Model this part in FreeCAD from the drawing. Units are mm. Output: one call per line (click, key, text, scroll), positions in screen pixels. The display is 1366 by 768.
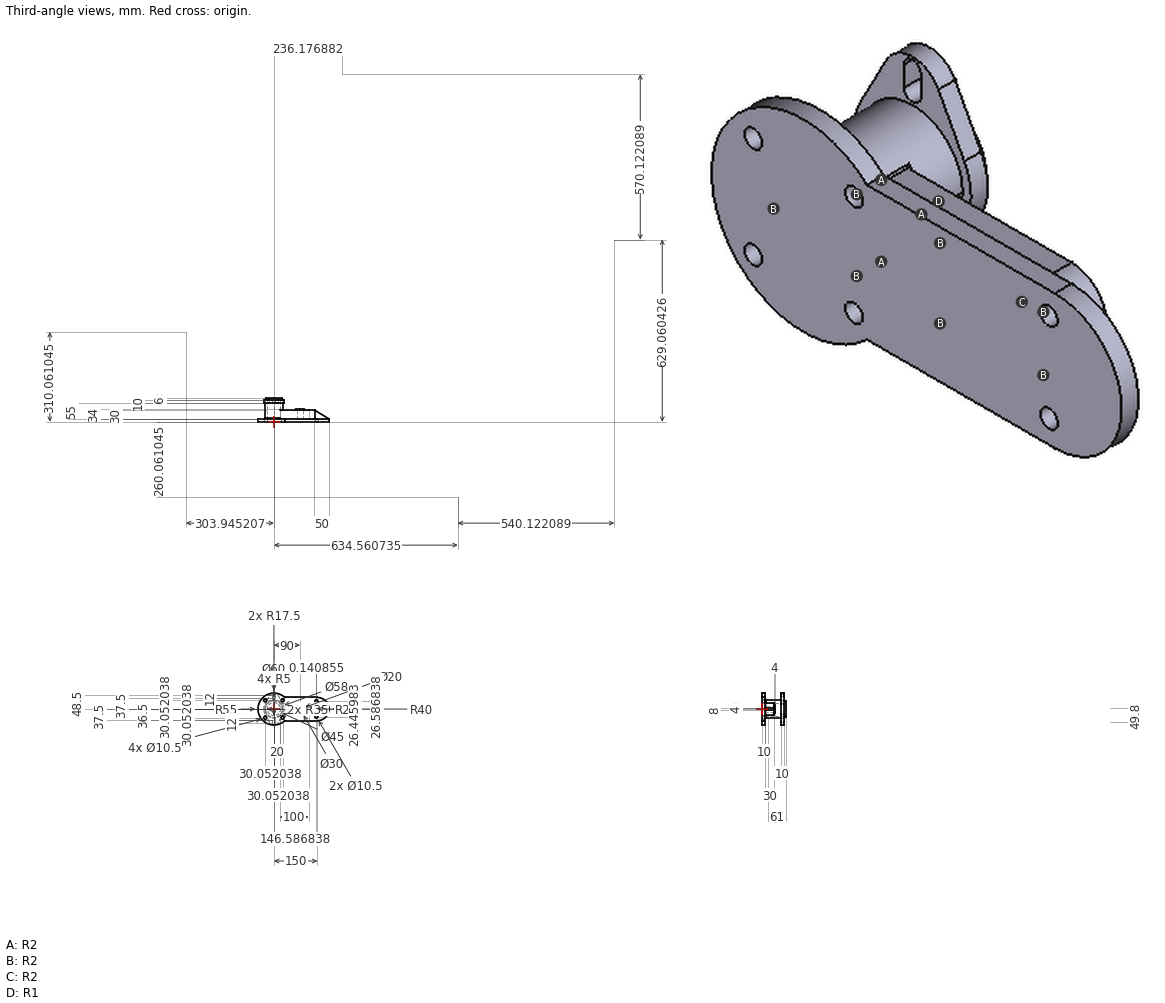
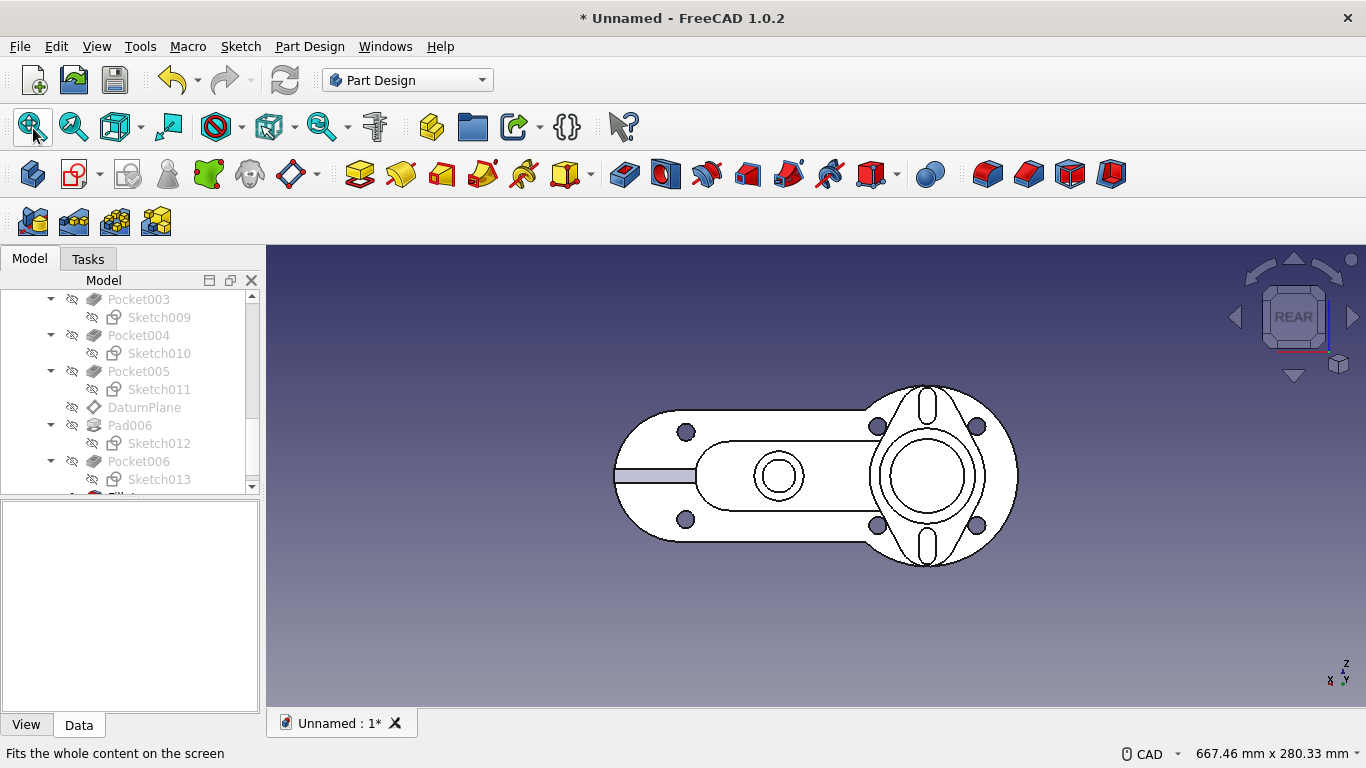
key(v)
key(f)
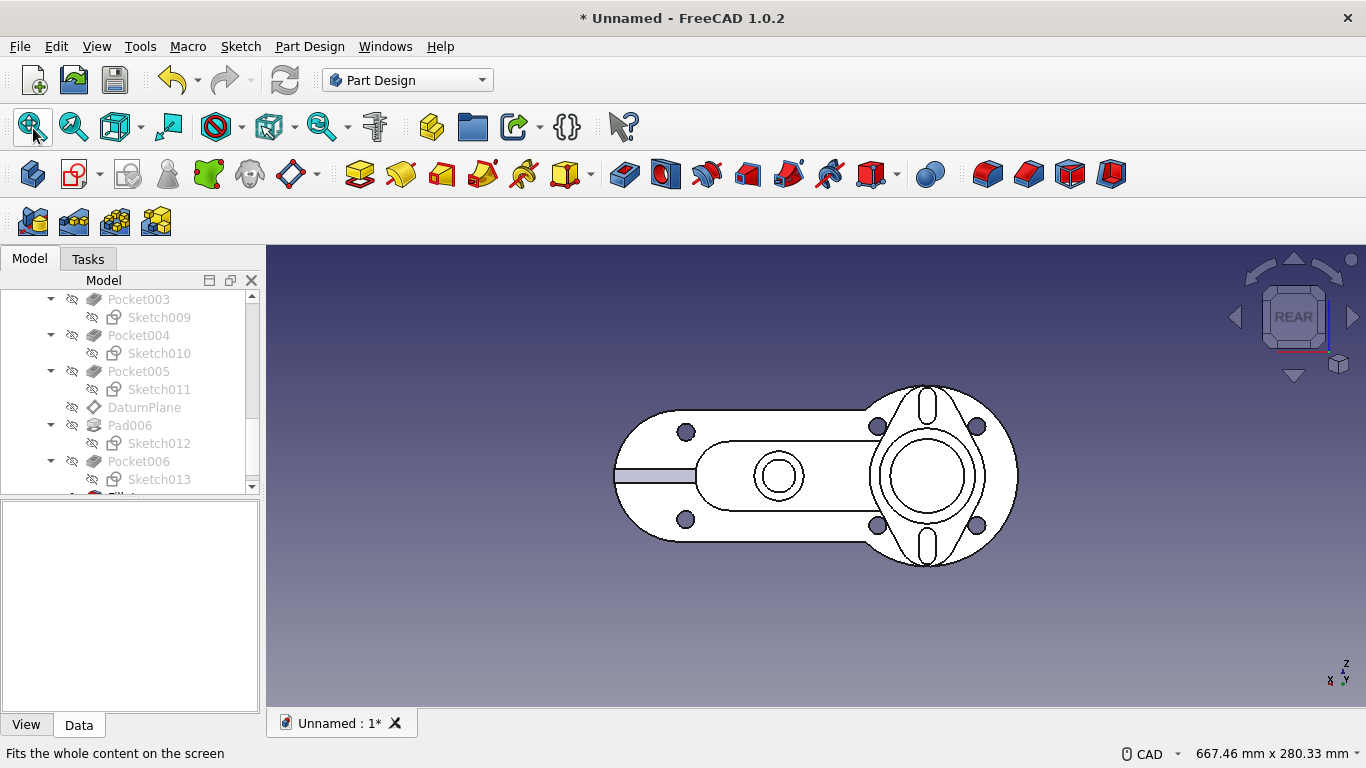
key(6)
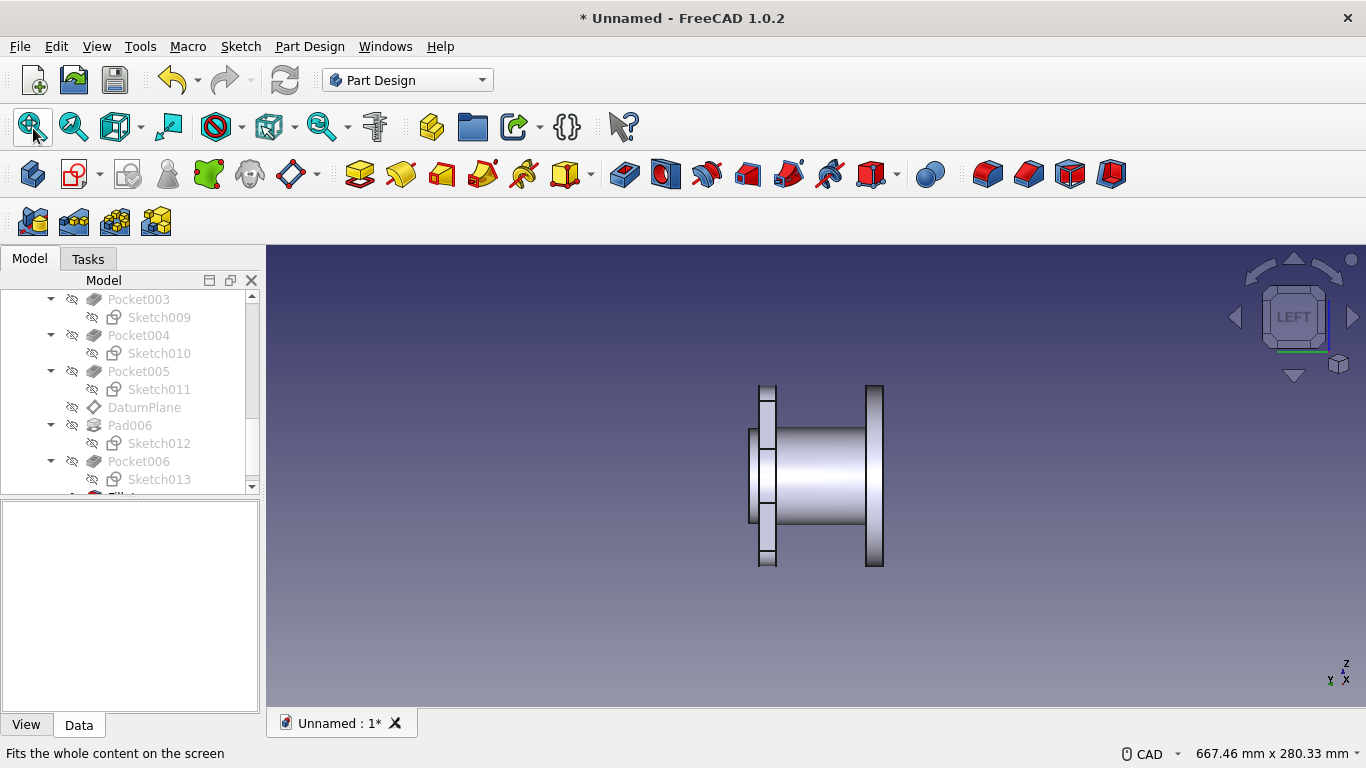
key(v)
key(f)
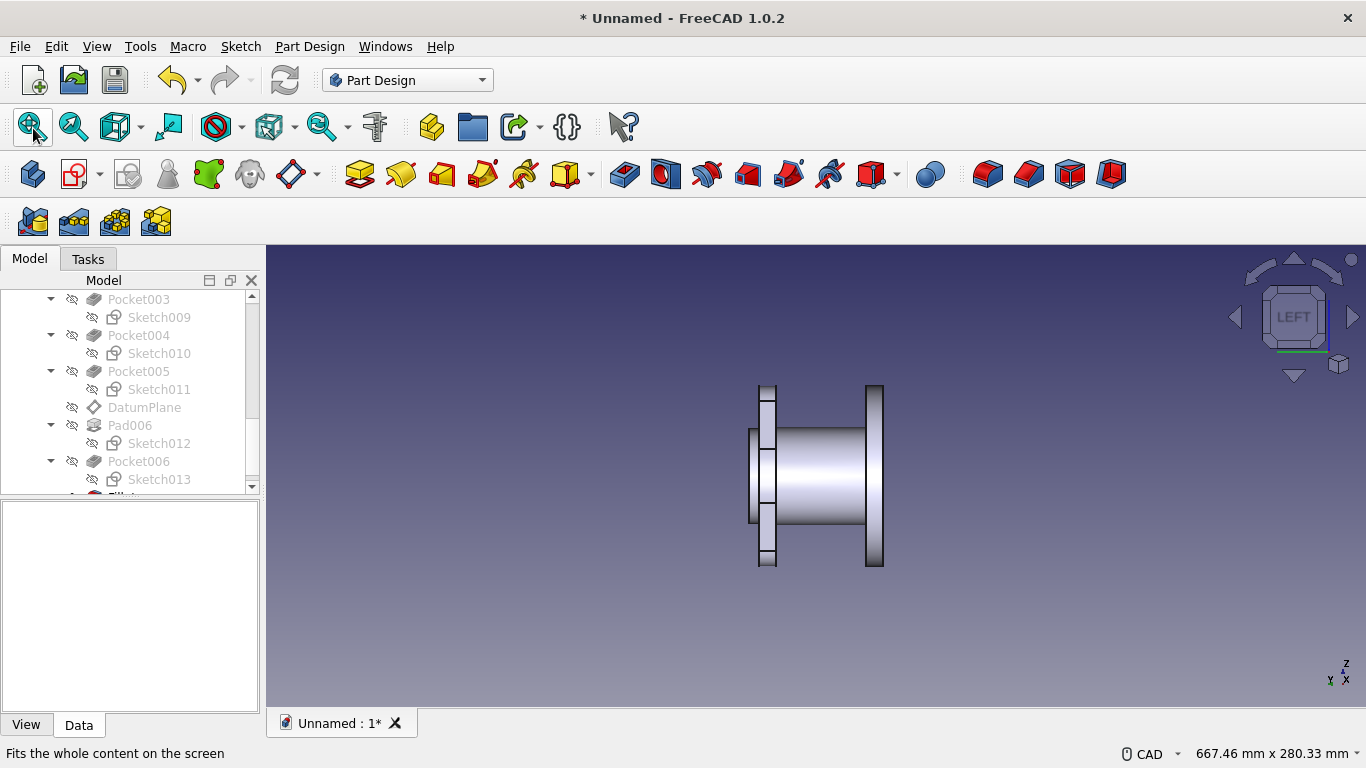
key(v)
key(3)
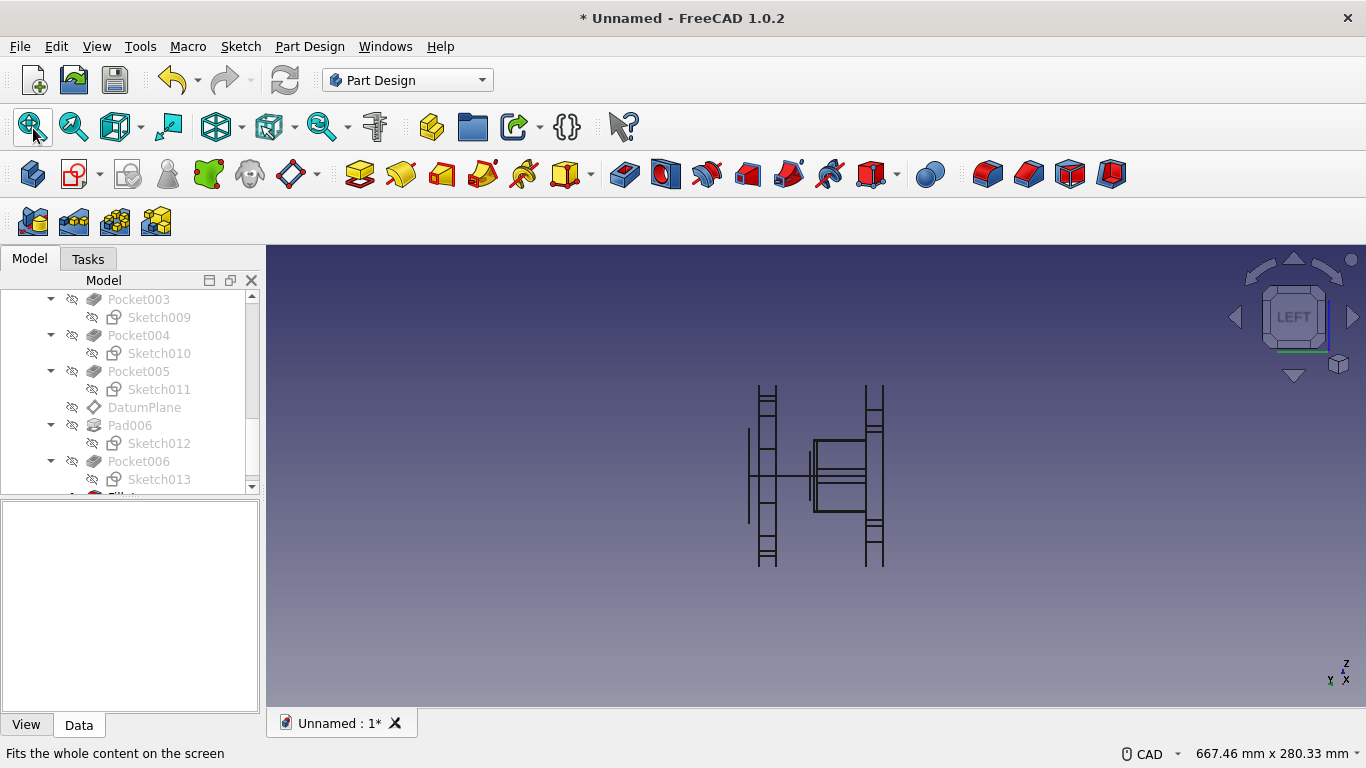
key(0)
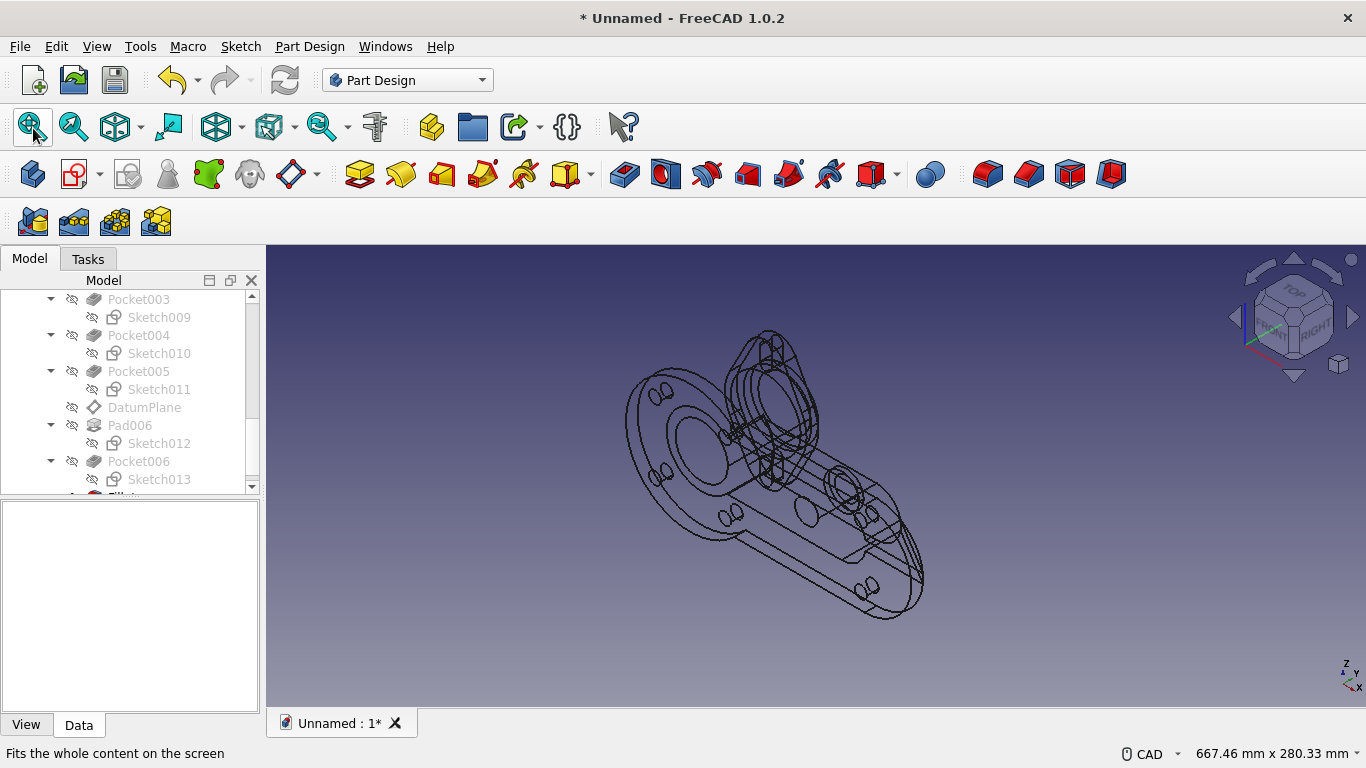
click(857, 562)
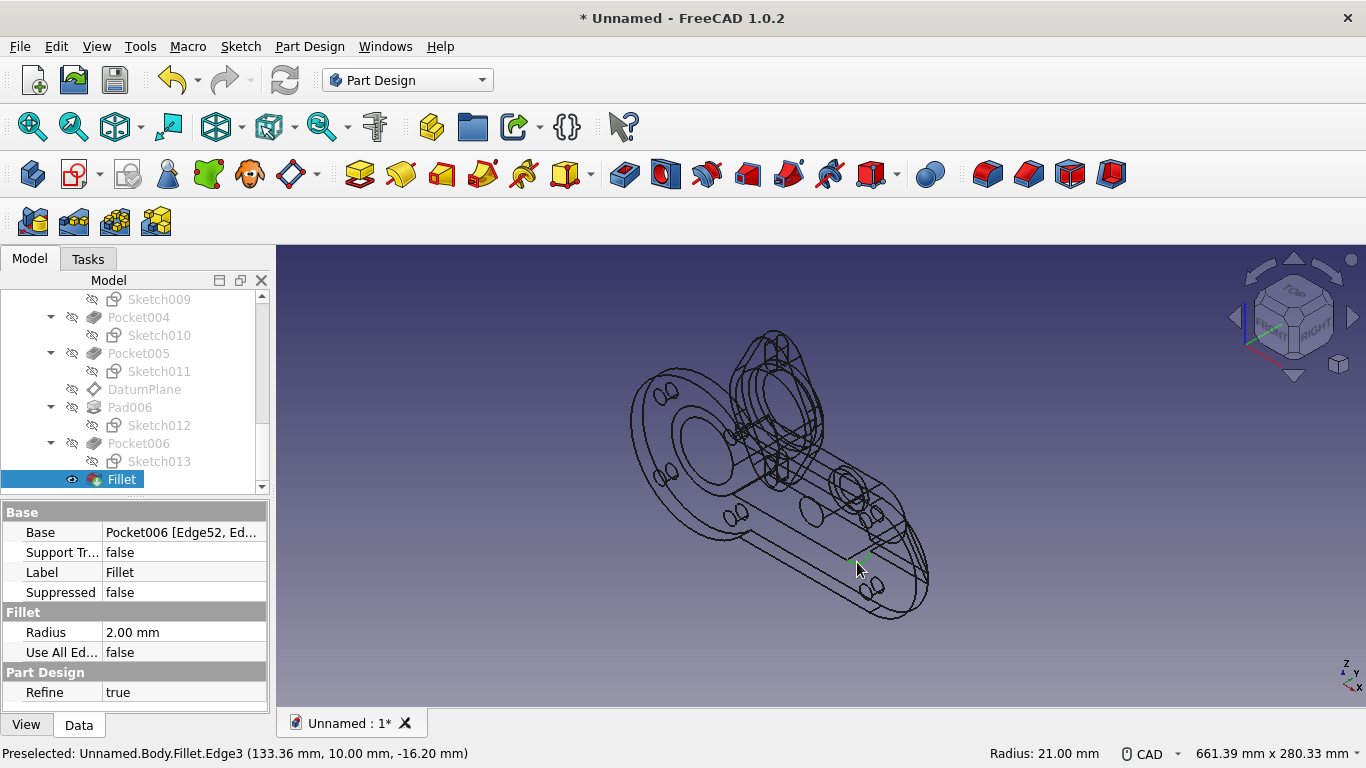
click(790, 470, ctrl)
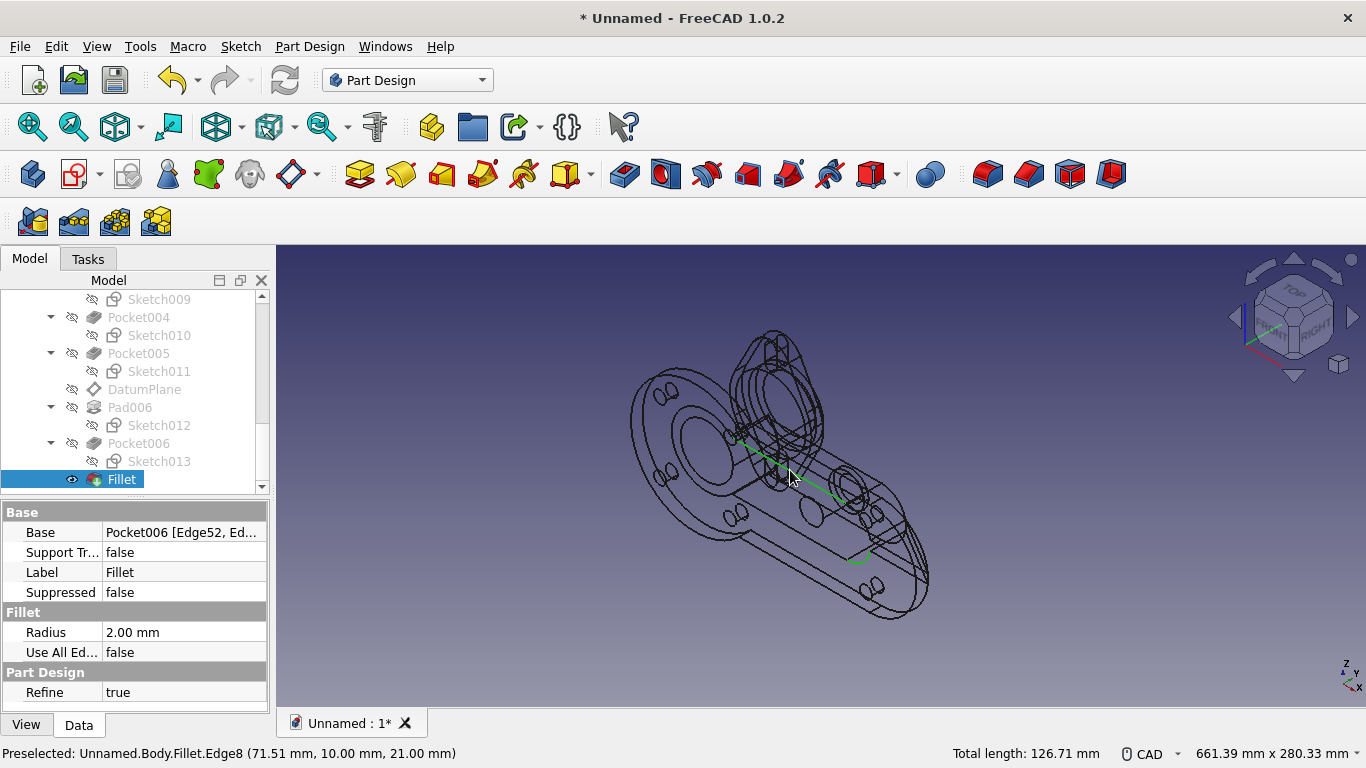
click(672, 430, ctrl)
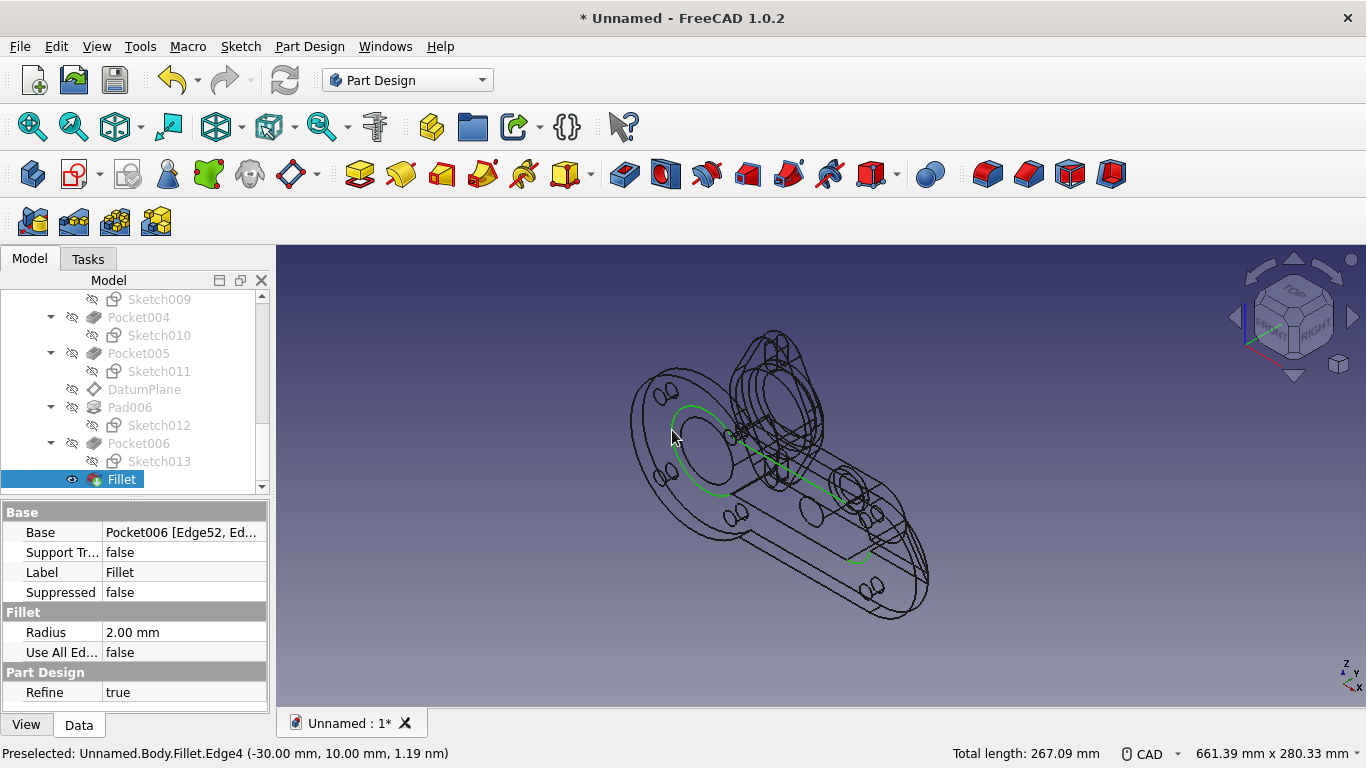
click(790, 526, ctrl)